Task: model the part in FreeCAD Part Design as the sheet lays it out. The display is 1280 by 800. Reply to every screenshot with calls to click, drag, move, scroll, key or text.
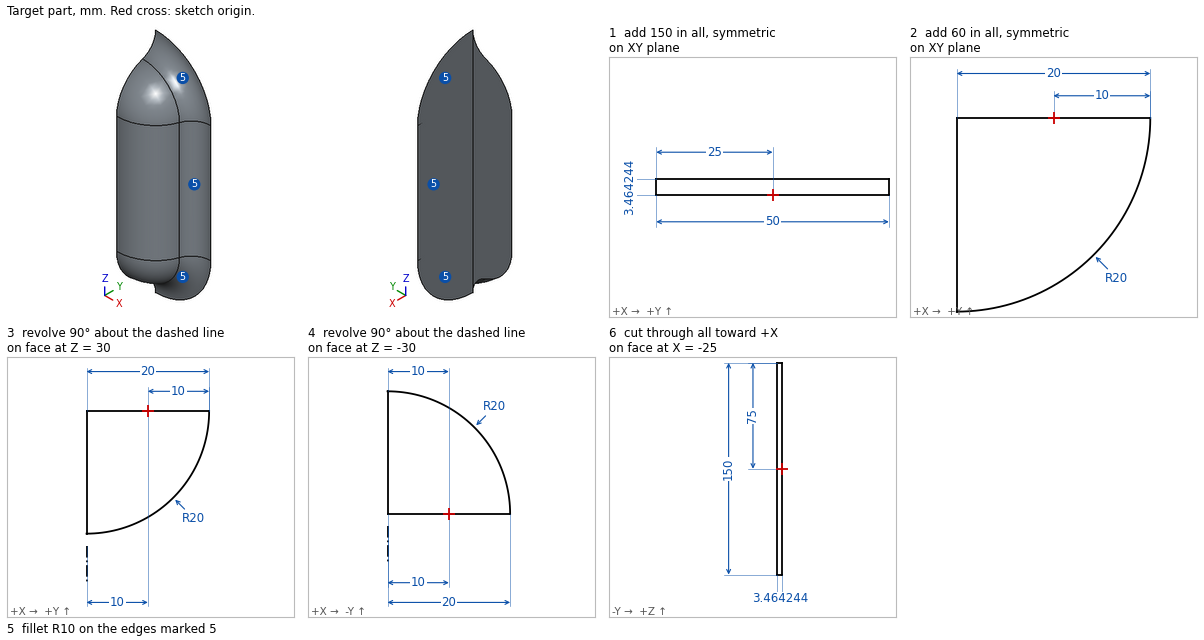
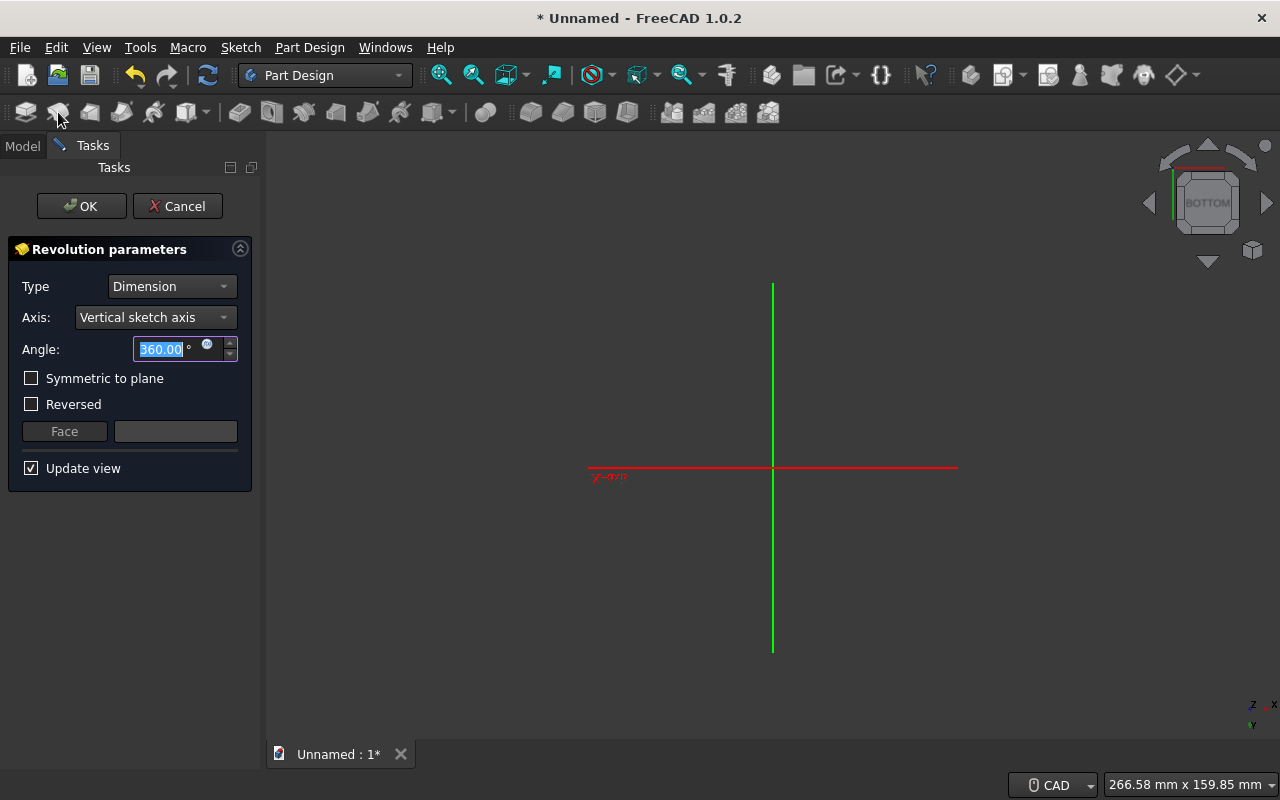
click(156, 318)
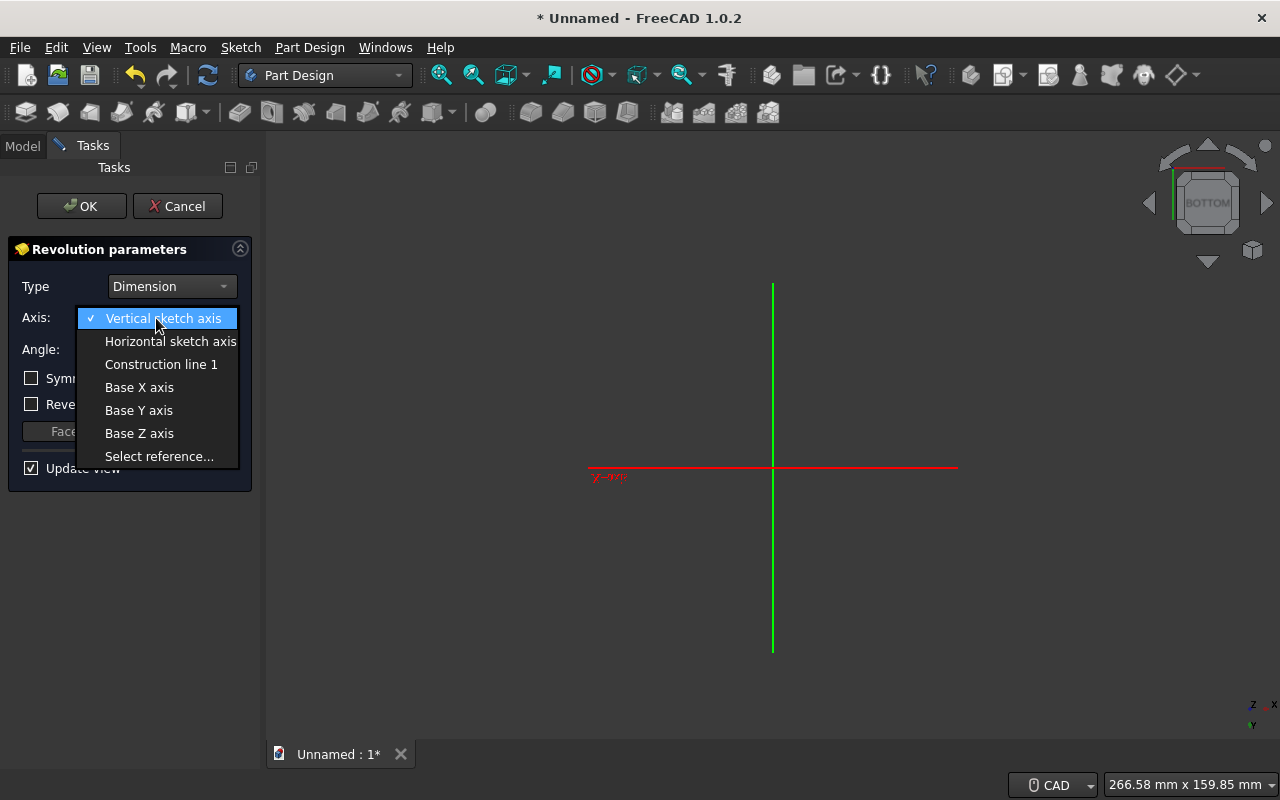
click(156, 364)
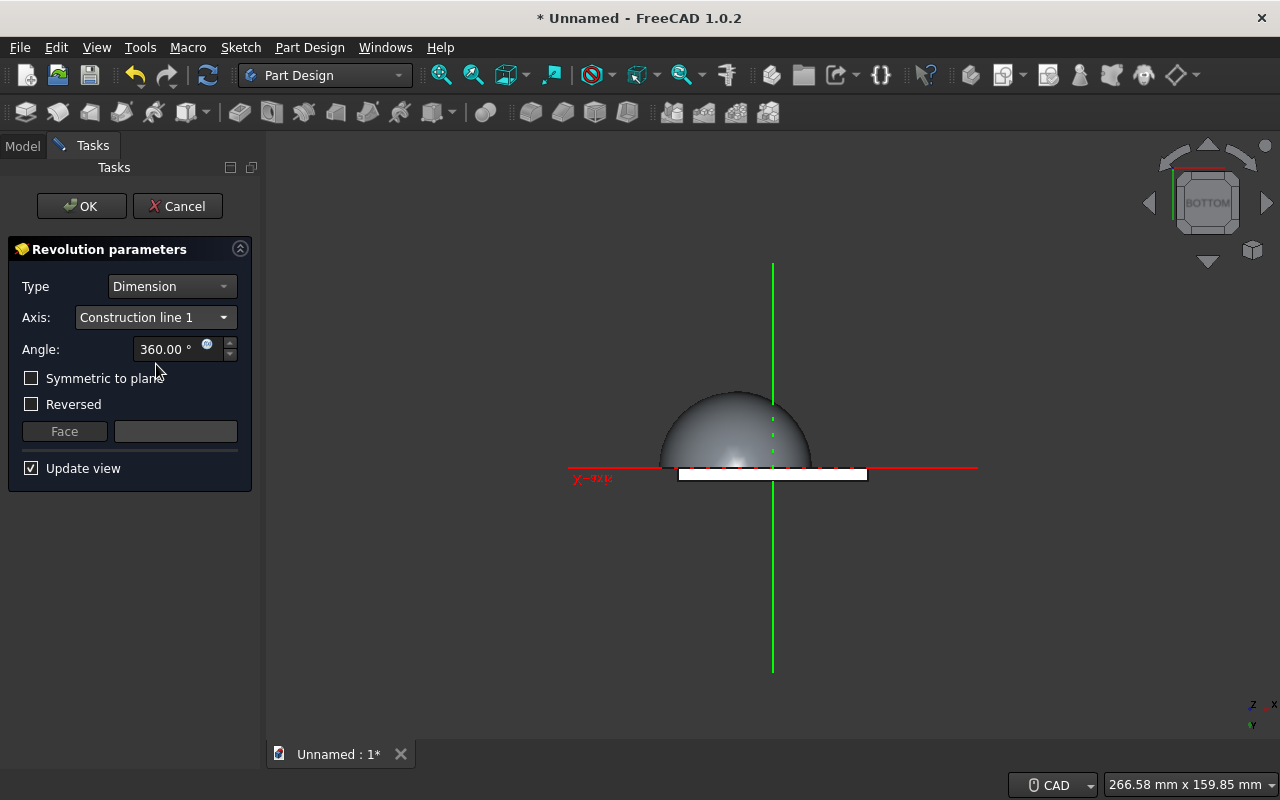
triple_click(178, 349)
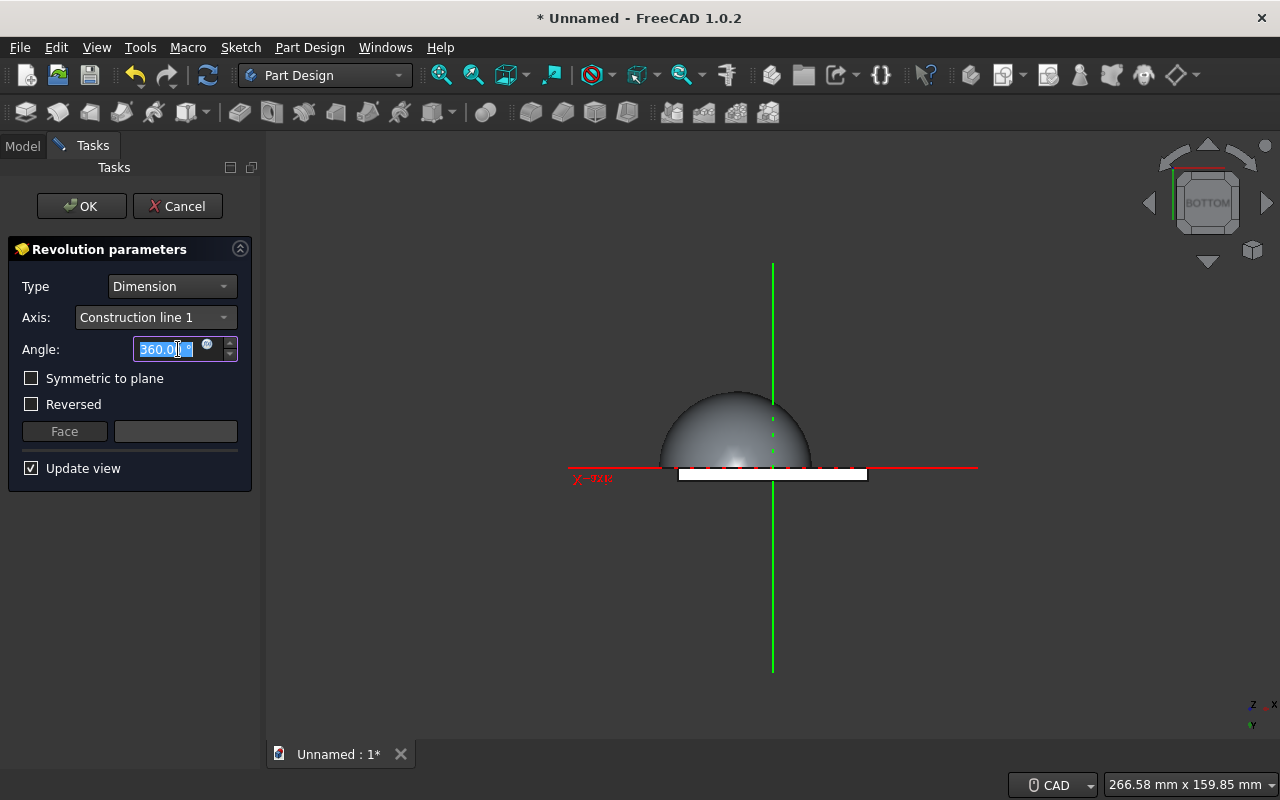
text(90)
key(Tab)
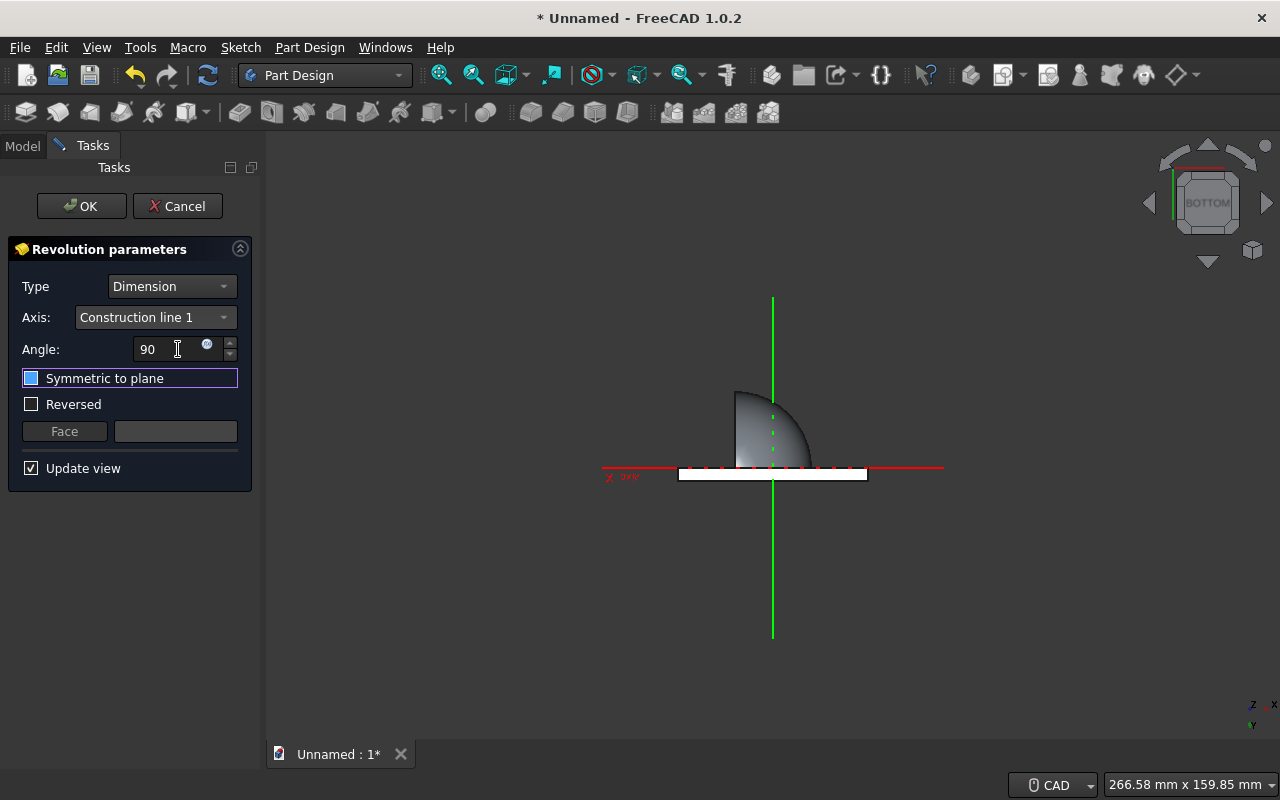
click(82, 206)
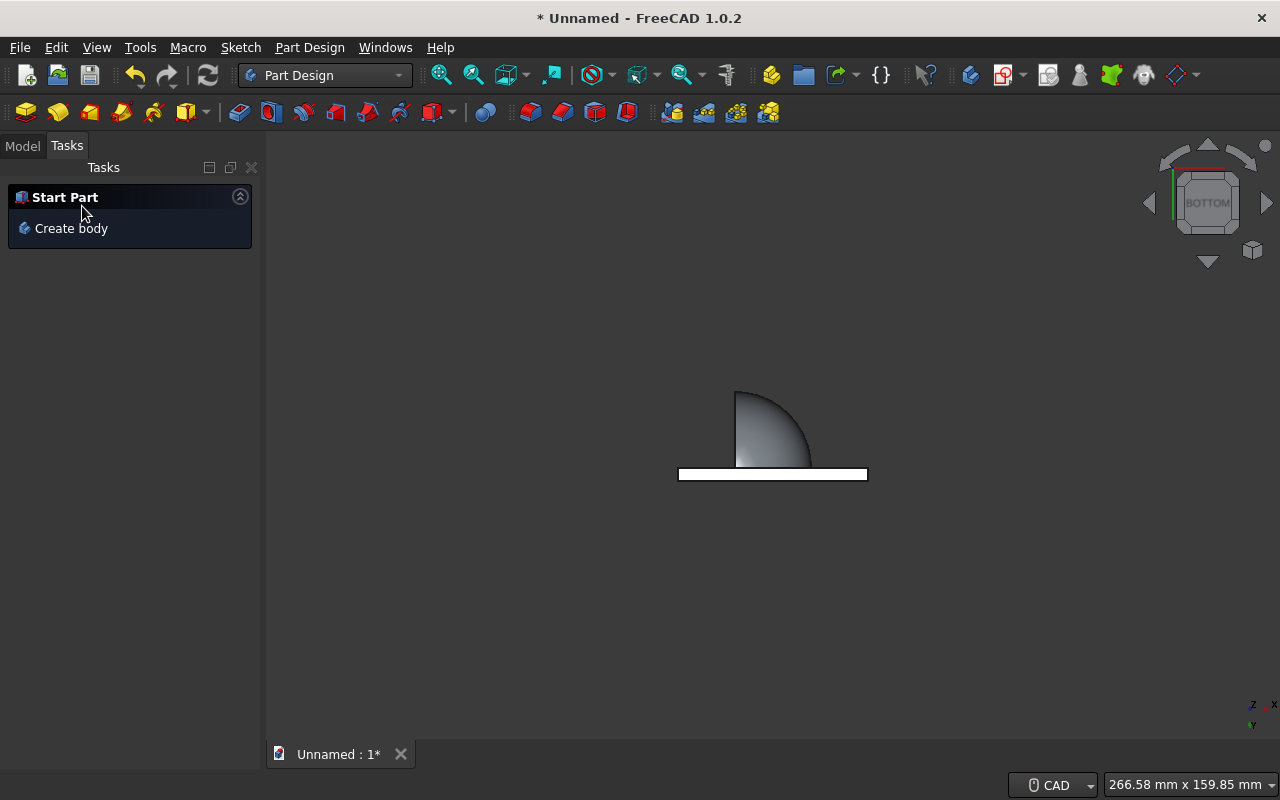
click(442, 76)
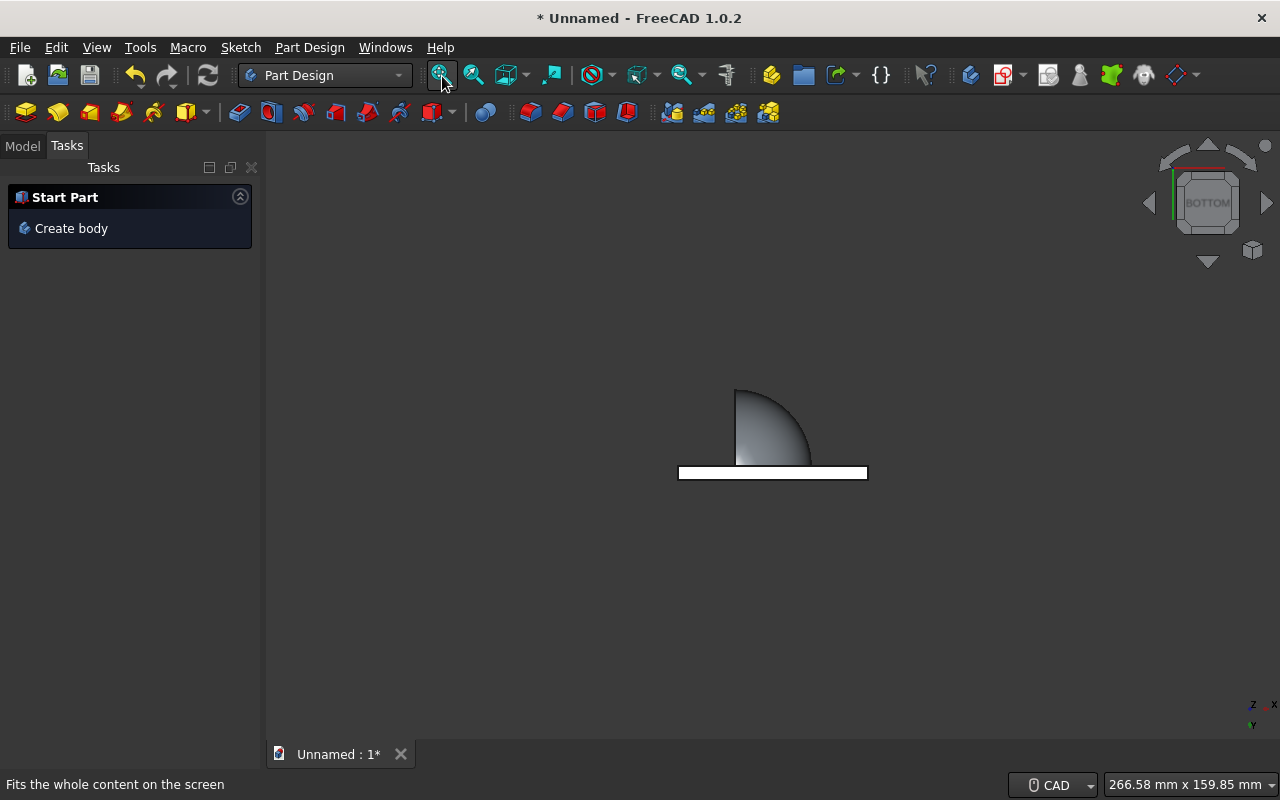
key(0)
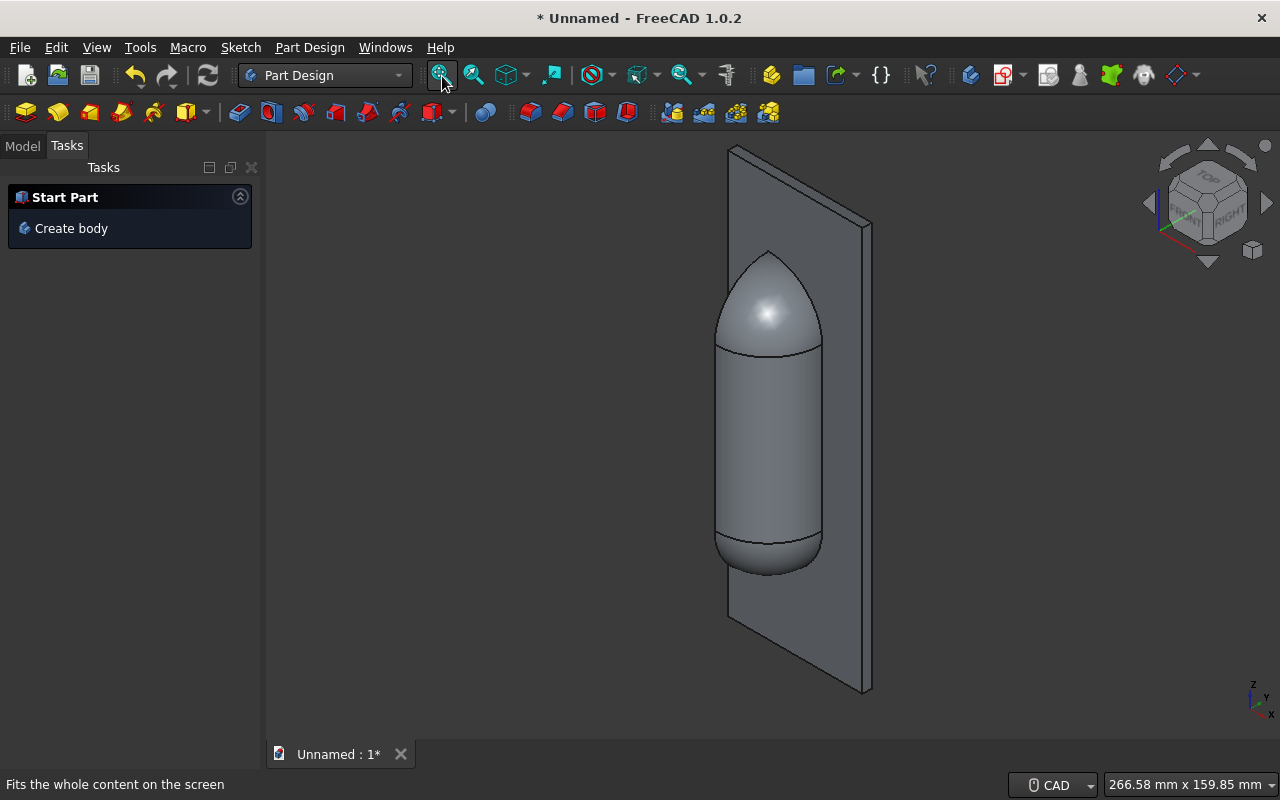
key(2)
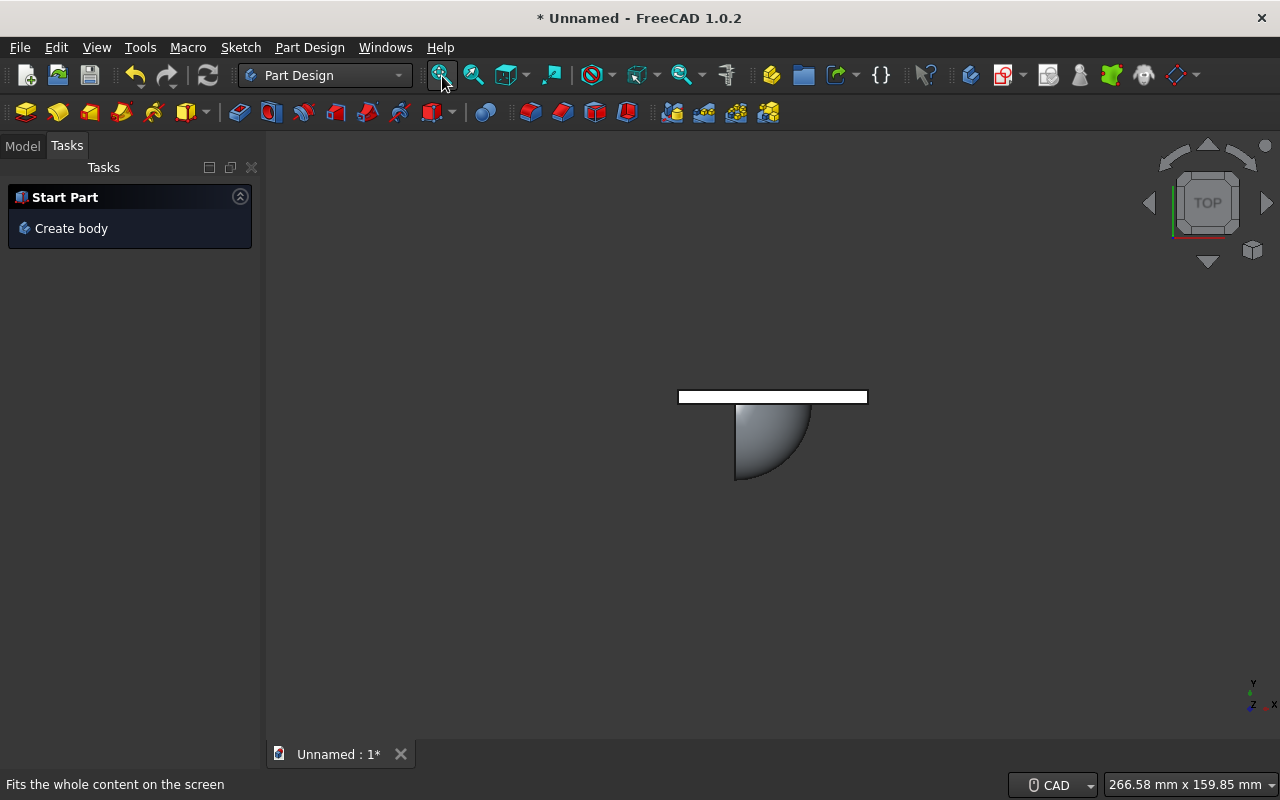
click(442, 76)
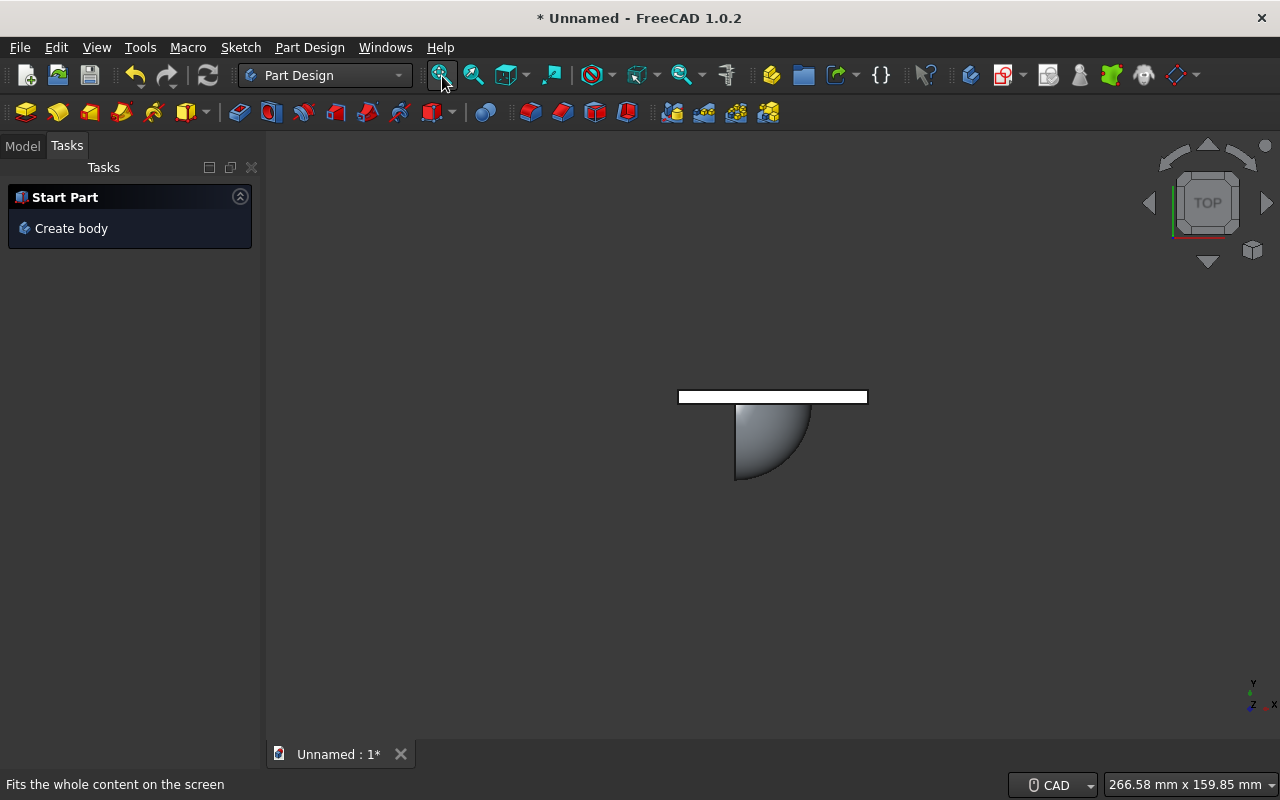
key(1)